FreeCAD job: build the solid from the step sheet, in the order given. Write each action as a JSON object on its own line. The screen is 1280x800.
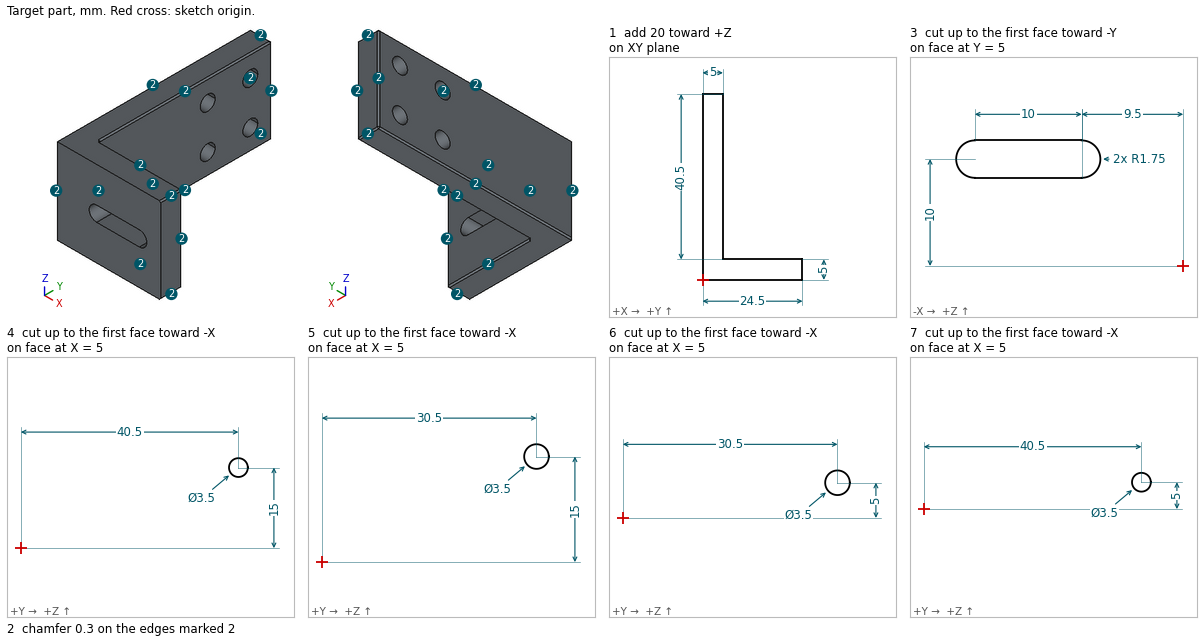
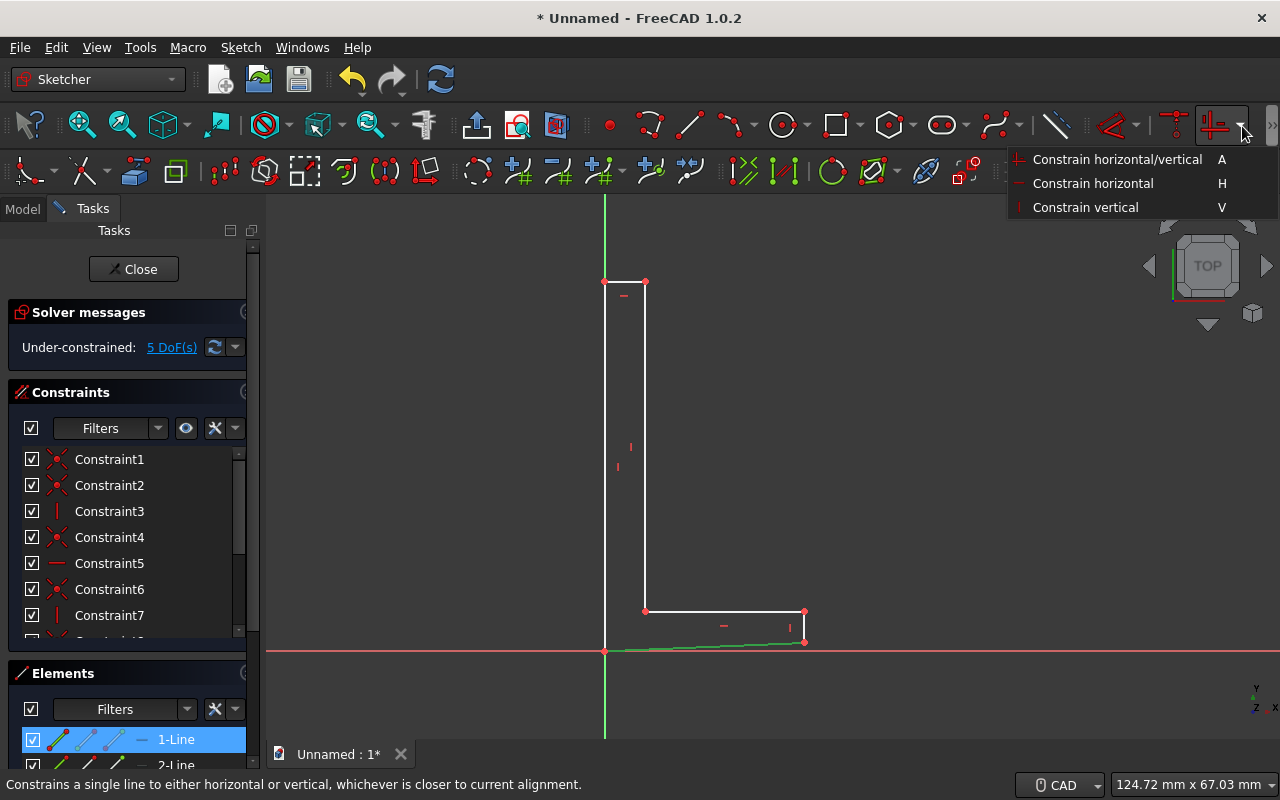
{"action": "left_click", "coordinate": [1143, 183]}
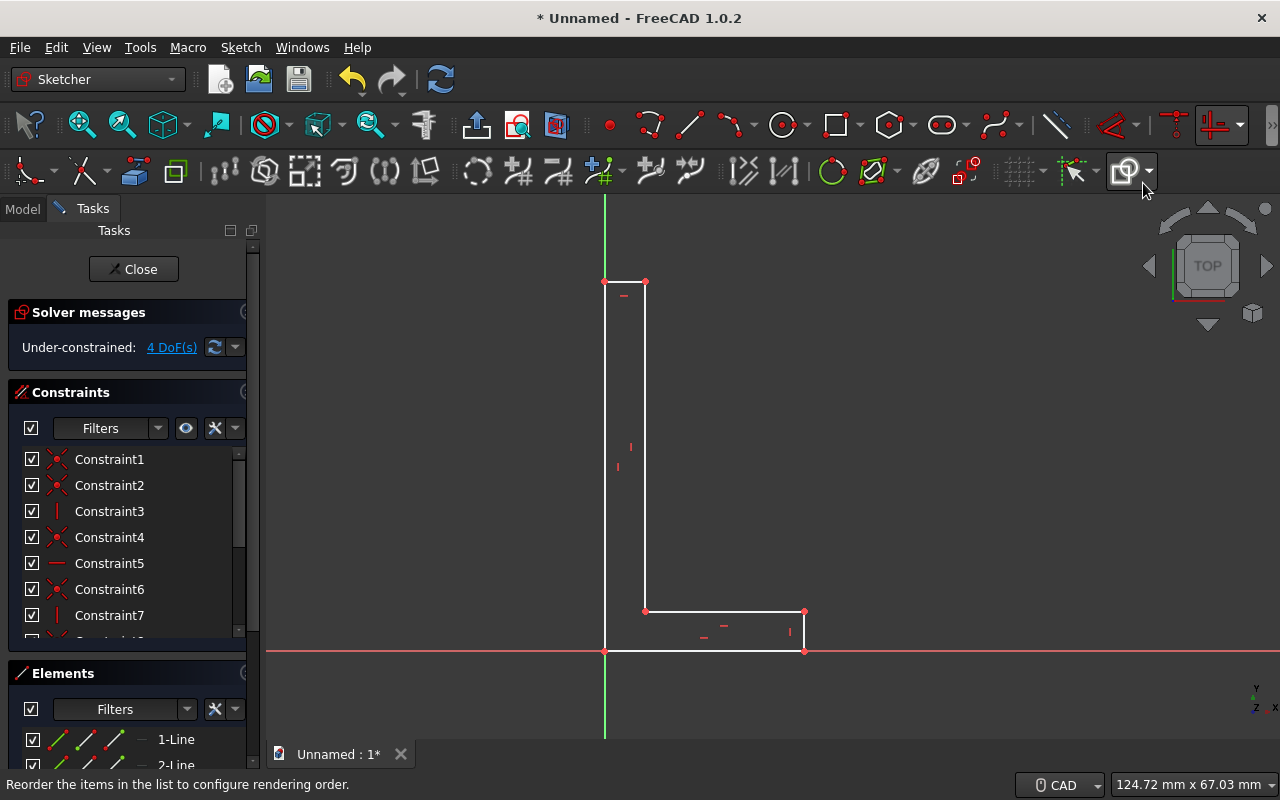
{"action": "left_click", "coordinate": [1112, 126]}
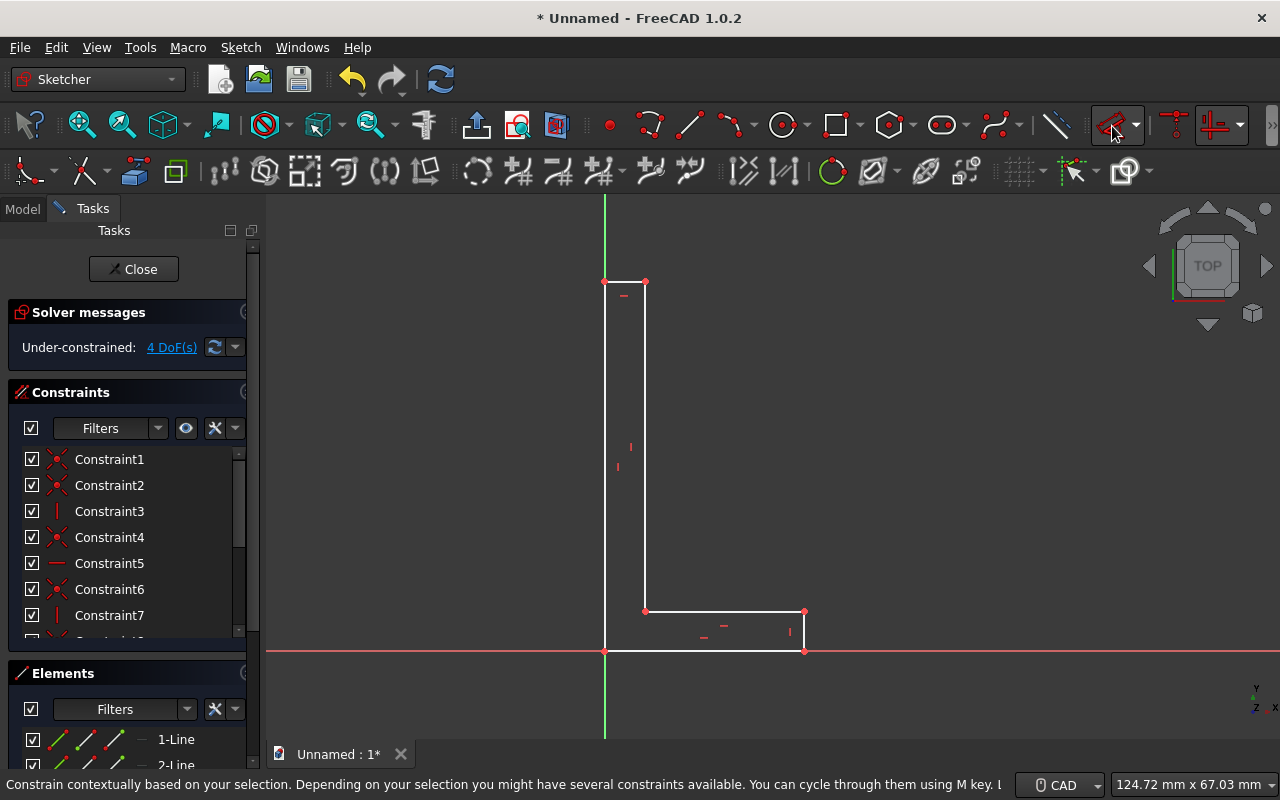
{"action": "left_click", "coordinate": [804, 640]}
{"action": "left_click", "coordinate": [838, 632]}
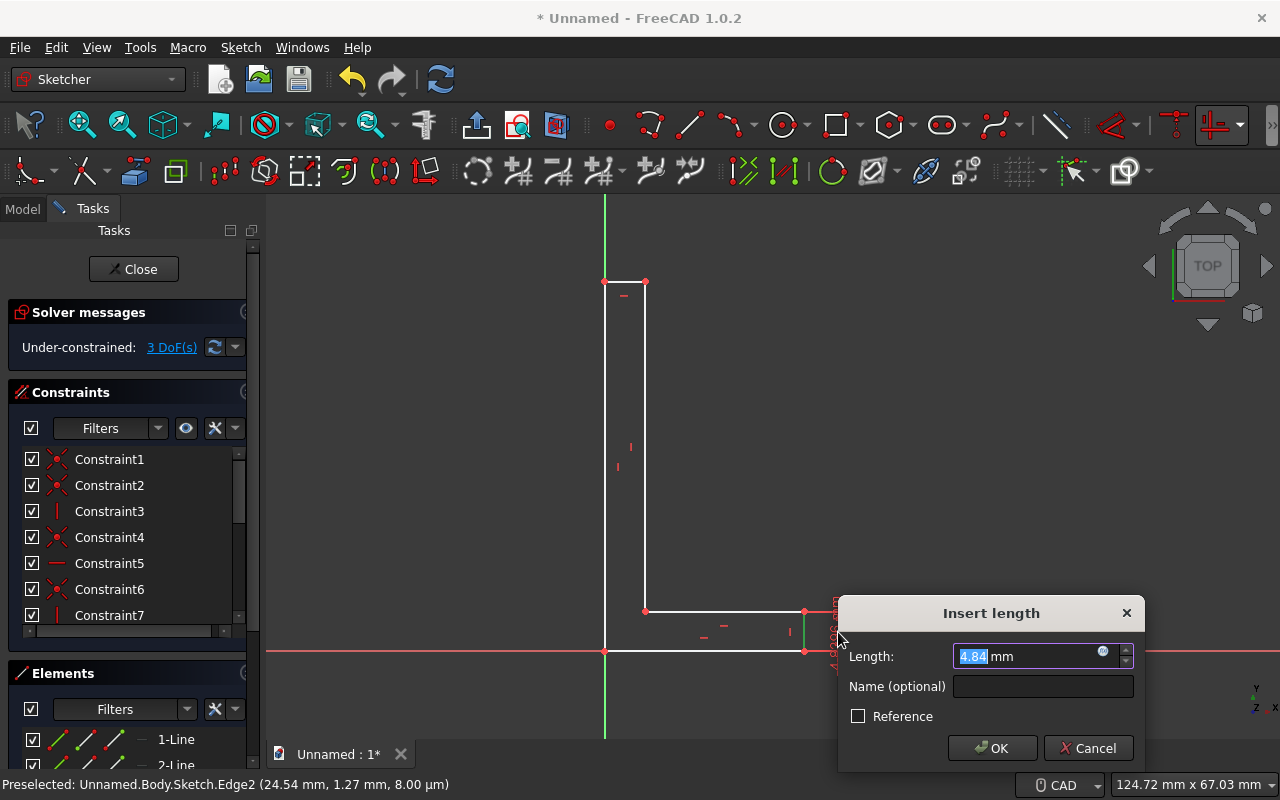
{"action": "type", "text": "5"}
{"action": "key", "text": "Return"}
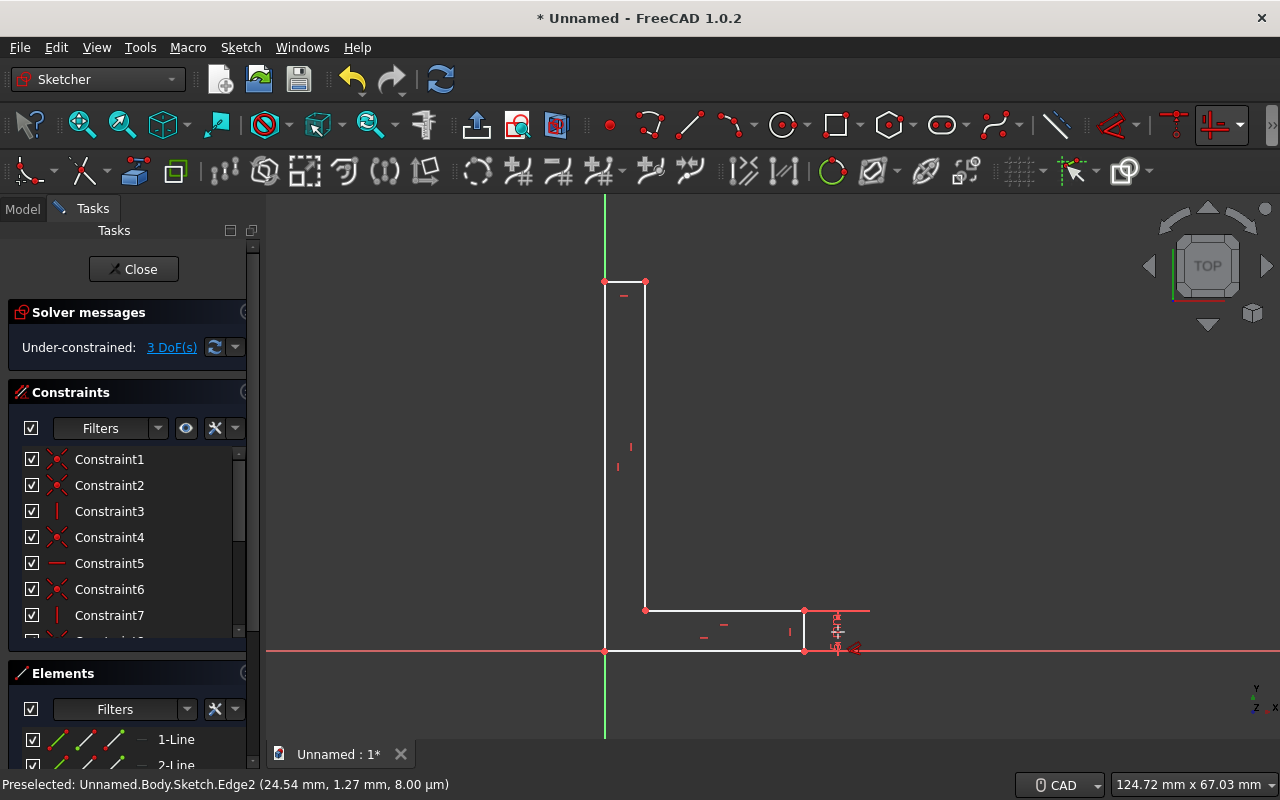
{"action": "left_click", "coordinate": [633, 282]}
{"action": "left_click", "coordinate": [625, 248]}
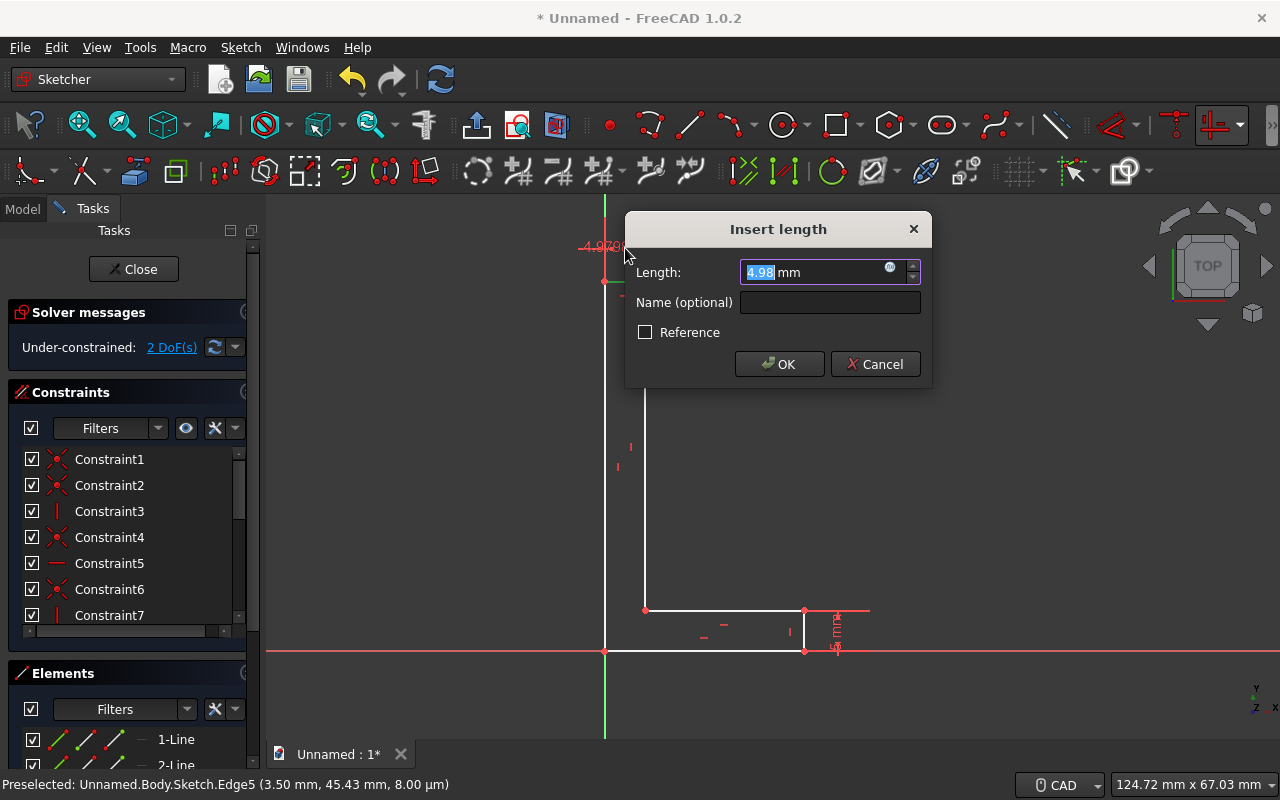
{"action": "type", "text": "5"}
{"action": "key", "text": "Return"}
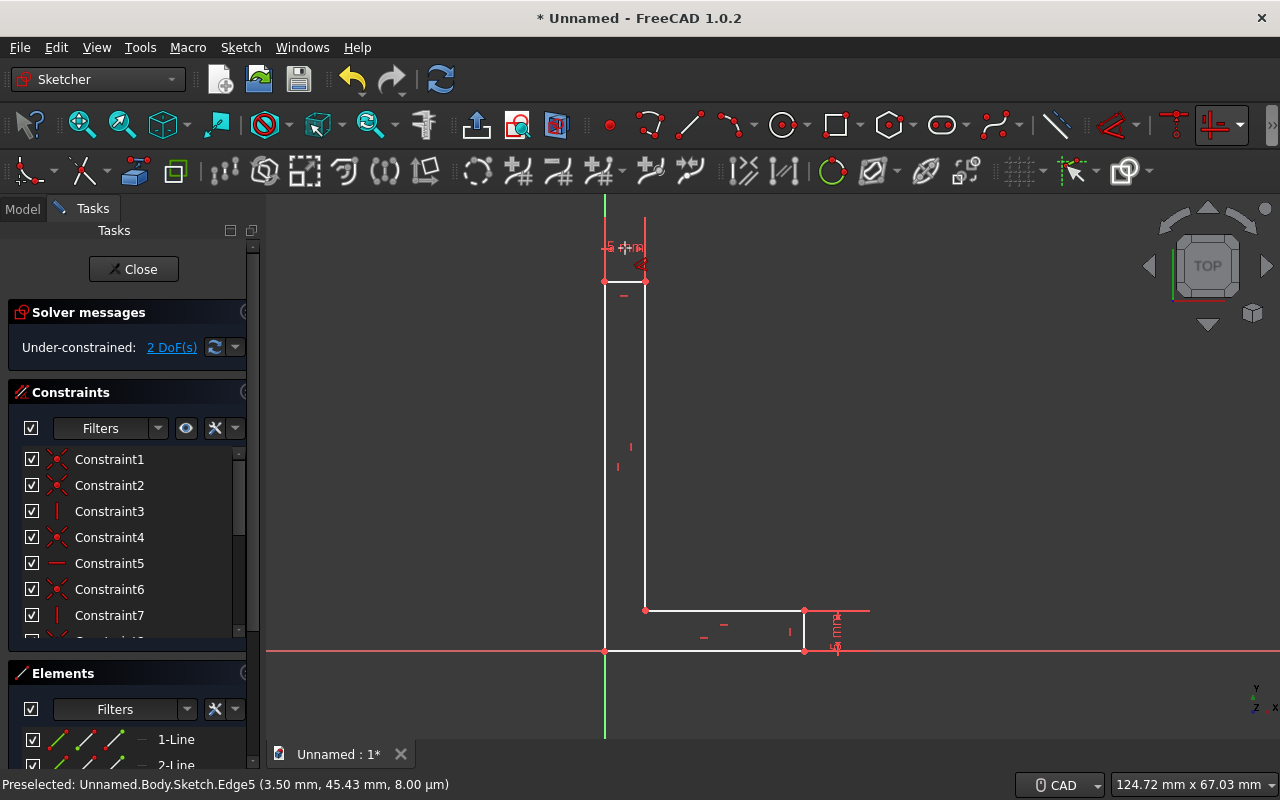
{"action": "left_click", "coordinate": [664, 651]}
{"action": "left_click", "coordinate": [704, 685]}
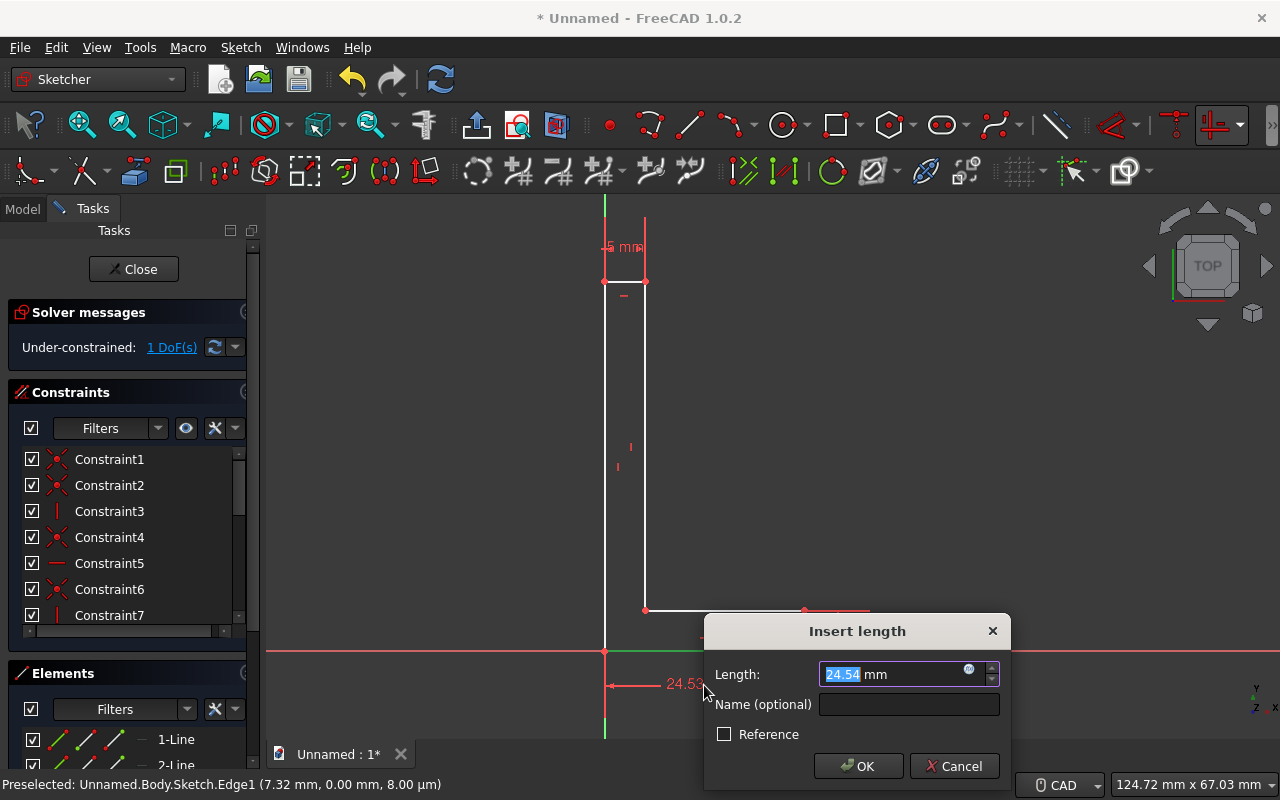
{"action": "type", "text": "24.5"}
{"action": "key", "text": "Return"}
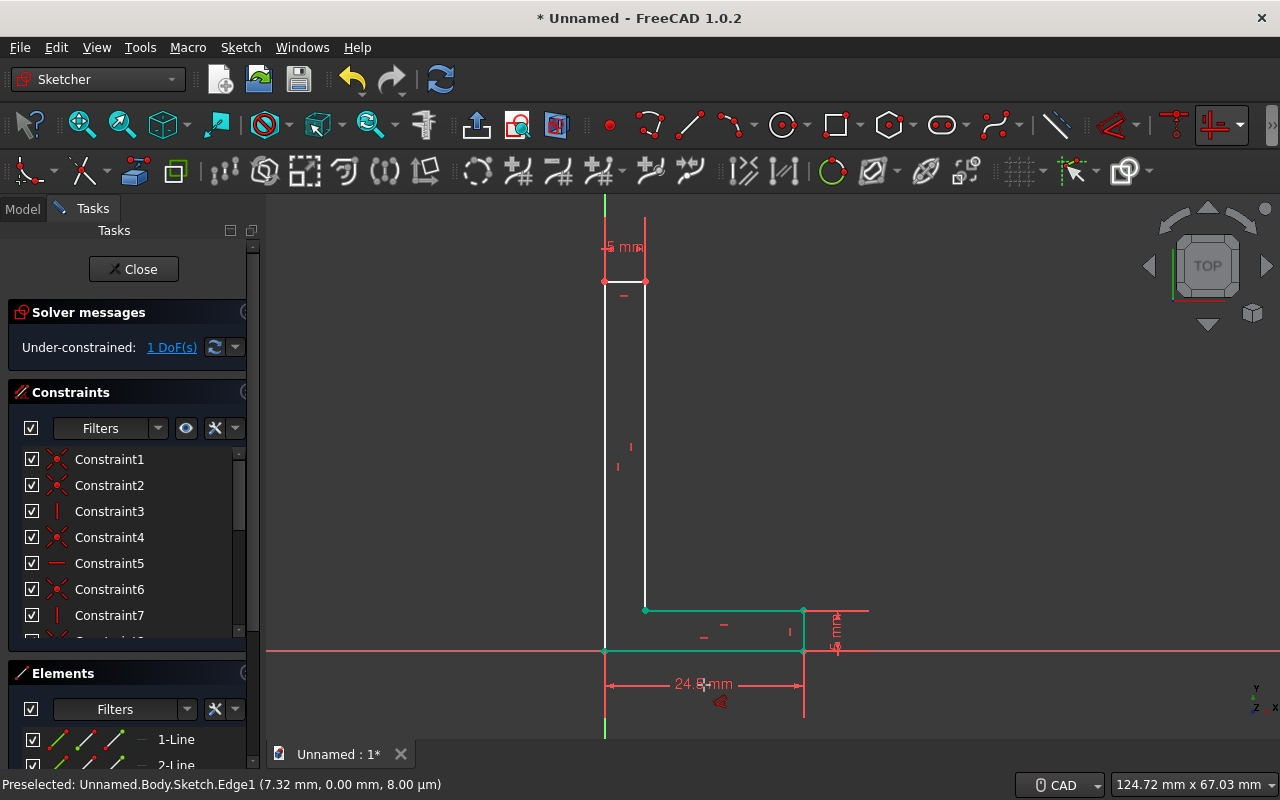
{"action": "left_click", "coordinate": [645, 512]}
{"action": "left_click", "coordinate": [679, 446]}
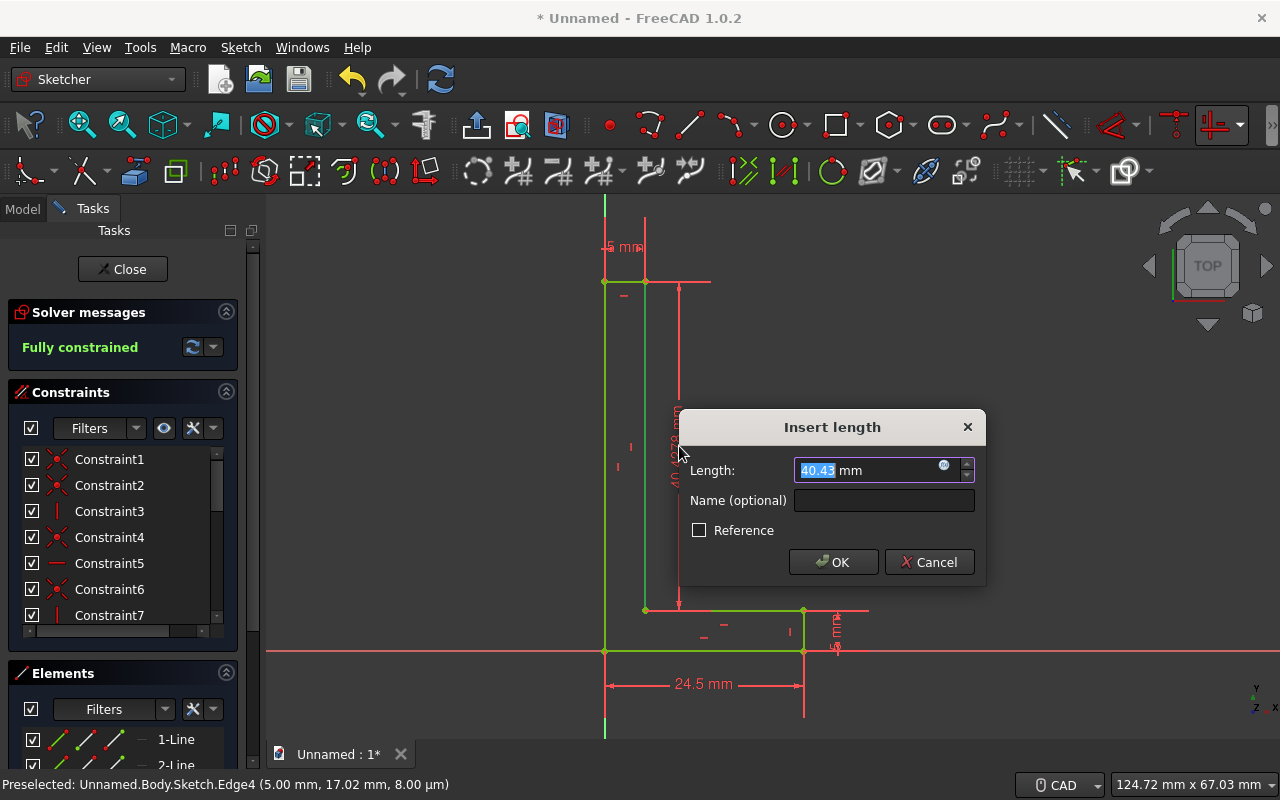
{"action": "type", "text": "40.5"}
{"action": "key", "text": "Return"}
{"action": "key", "text": "Escape"}